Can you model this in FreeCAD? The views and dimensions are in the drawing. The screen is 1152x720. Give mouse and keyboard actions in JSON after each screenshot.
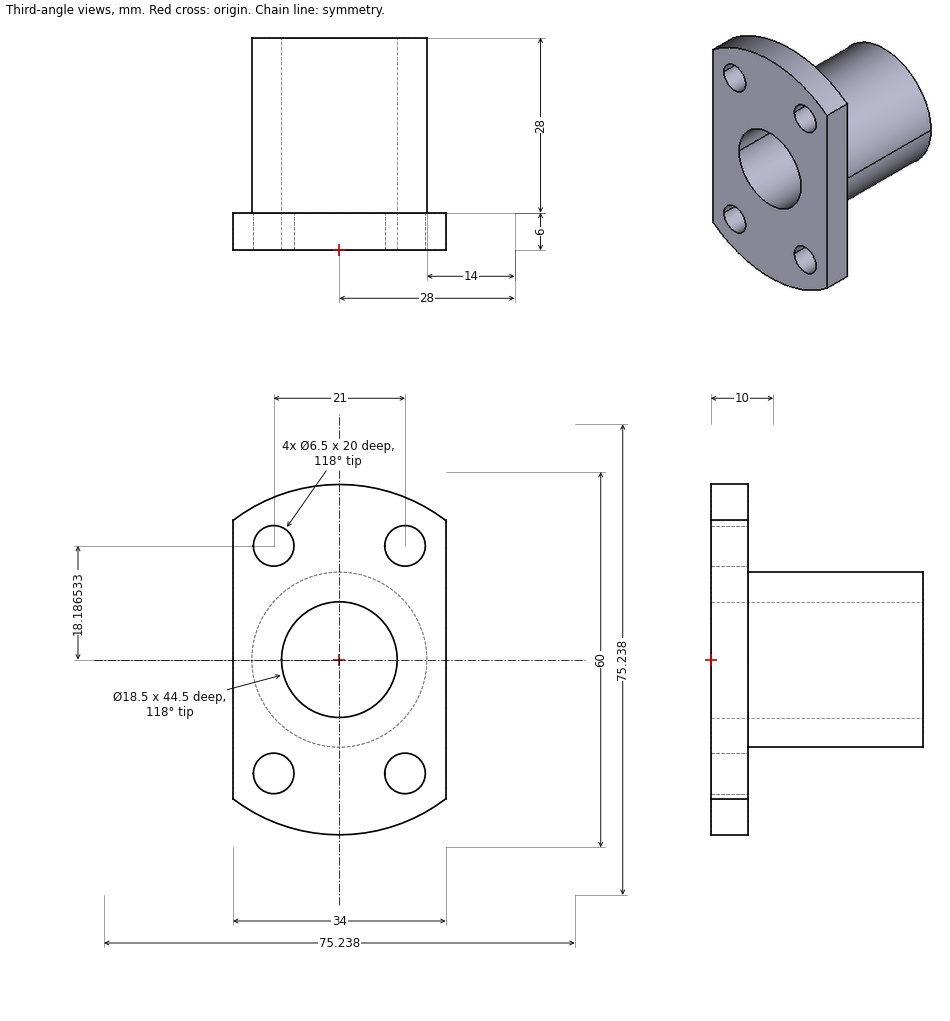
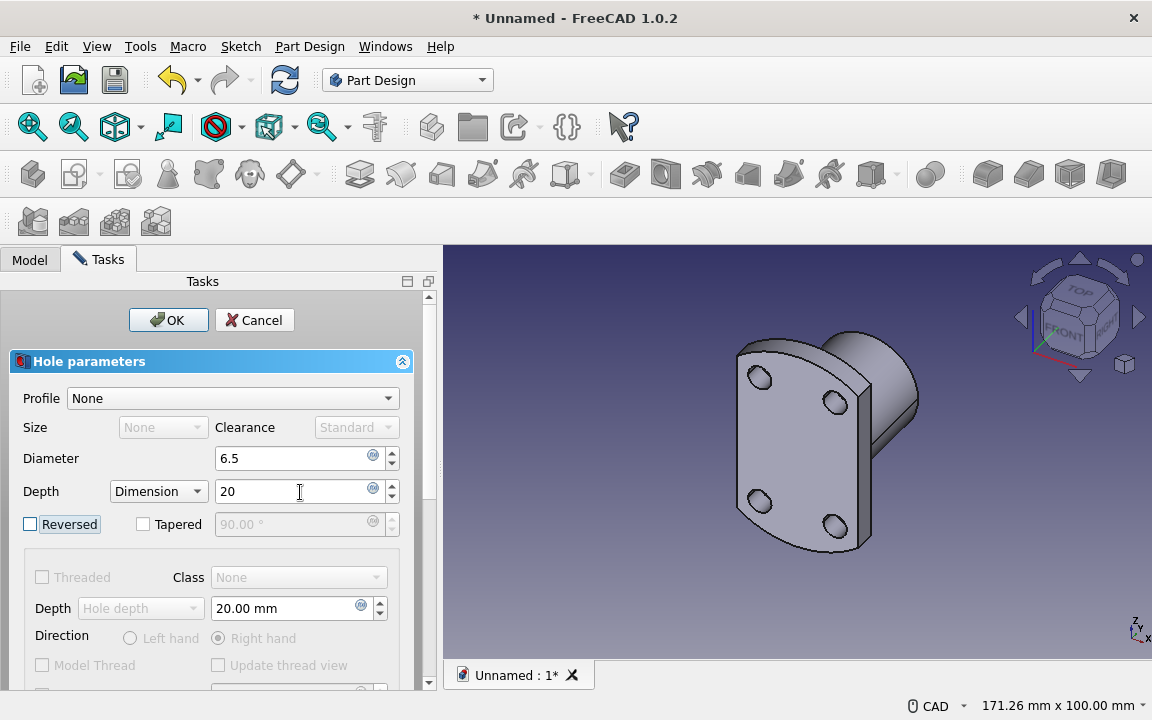
{"action": "left_click", "coordinate": [169, 320]}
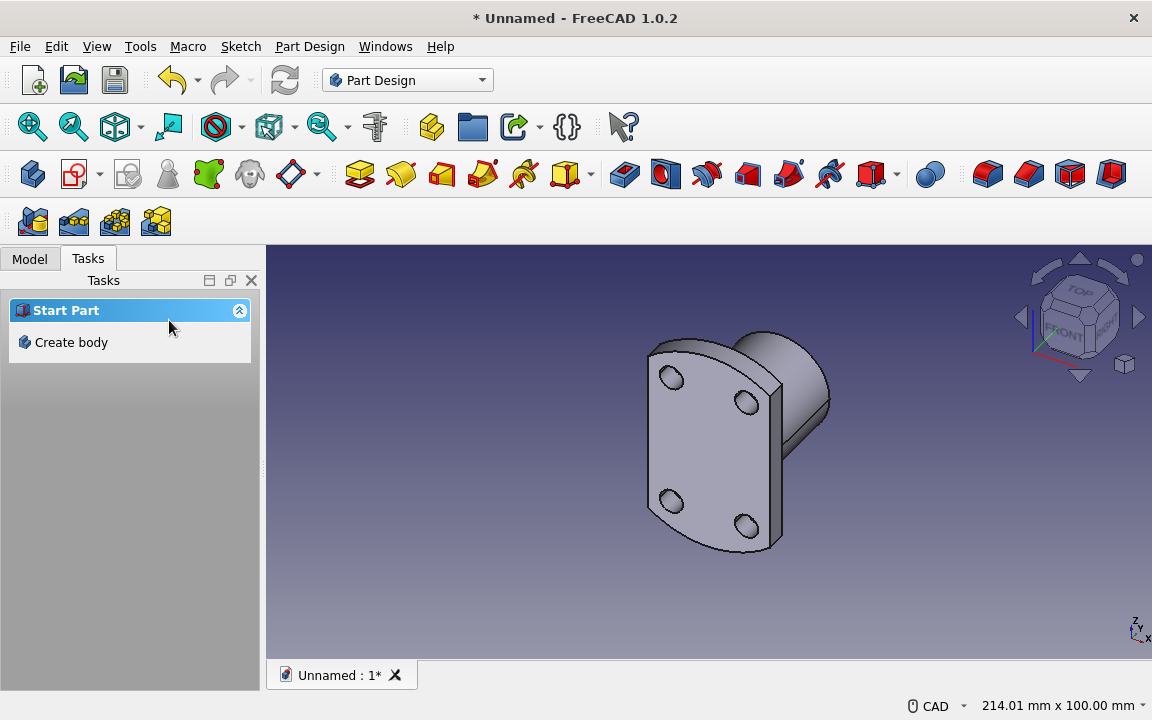
{"action": "left_click", "coordinate": [709, 451]}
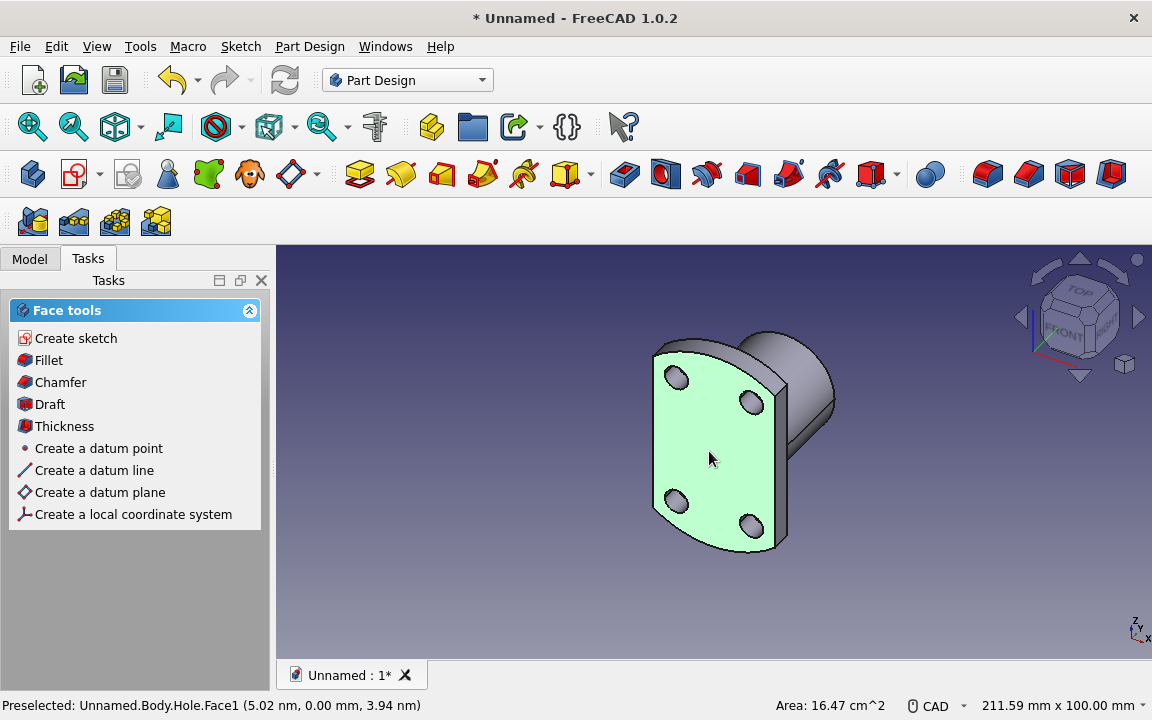
{"action": "left_click", "coordinate": [74, 174]}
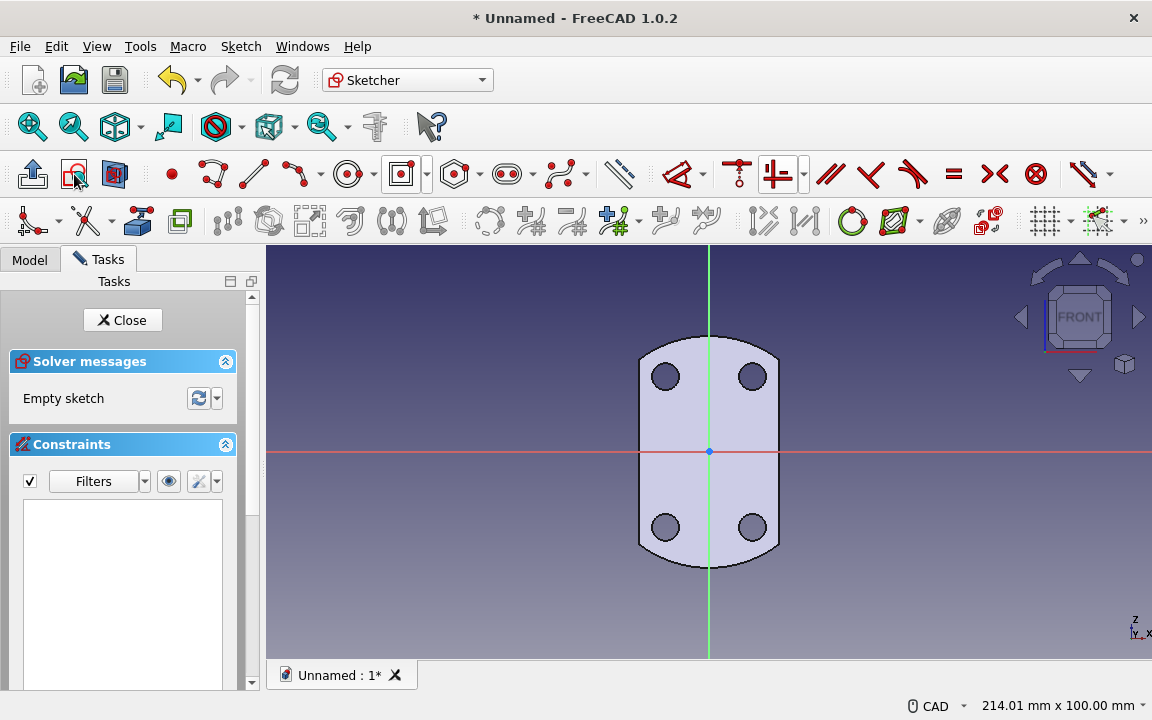
{"action": "scroll", "coordinate": [739, 452], "scroll_direction": "up", "scroll_amount": 6}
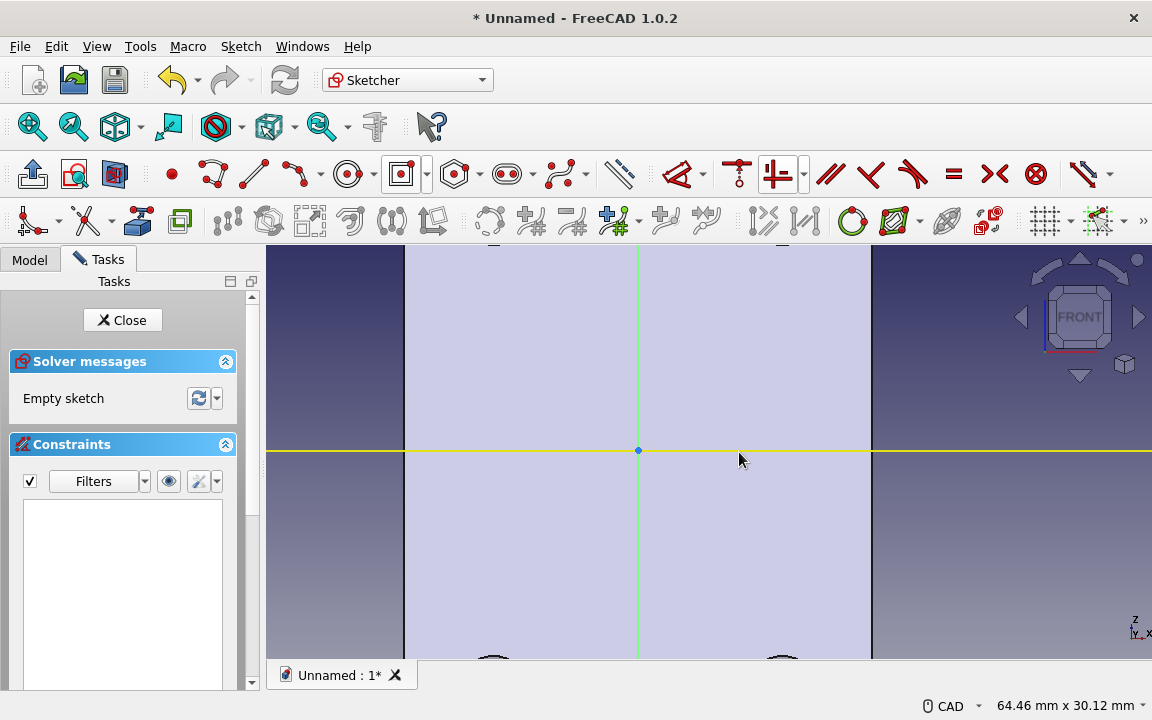
{"action": "left_click", "coordinate": [348, 174]}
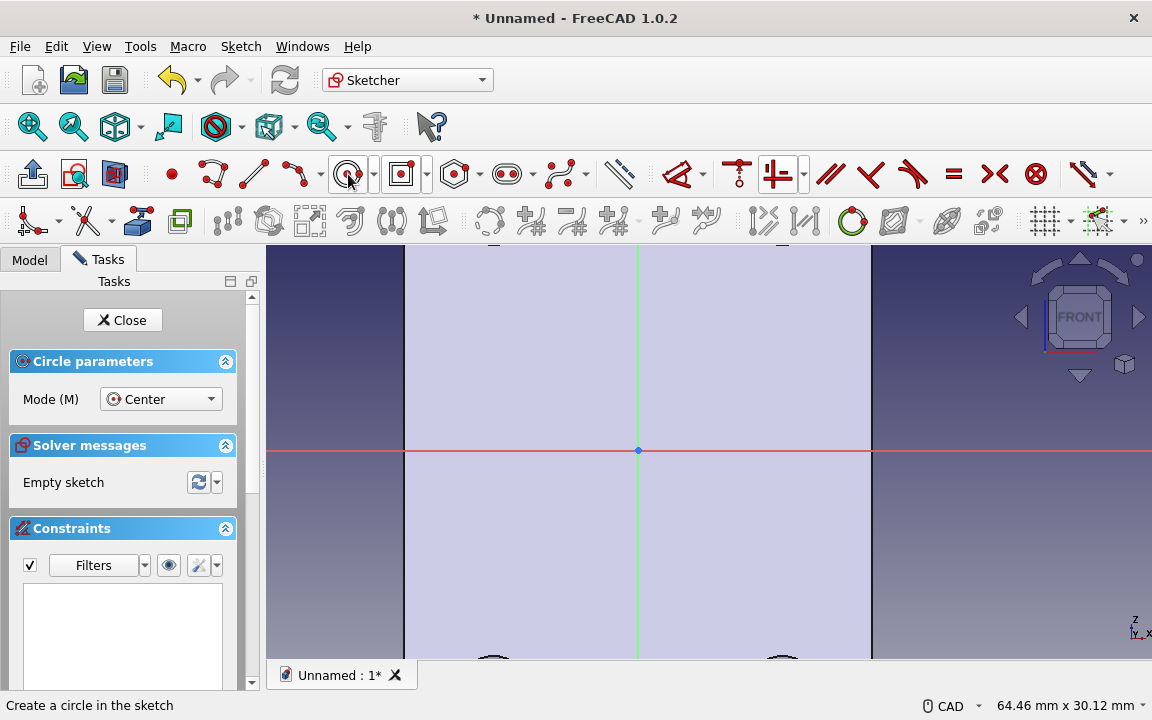
{"action": "left_click", "coordinate": [638, 451]}
{"action": "mouse_move", "coordinate": [728, 361]}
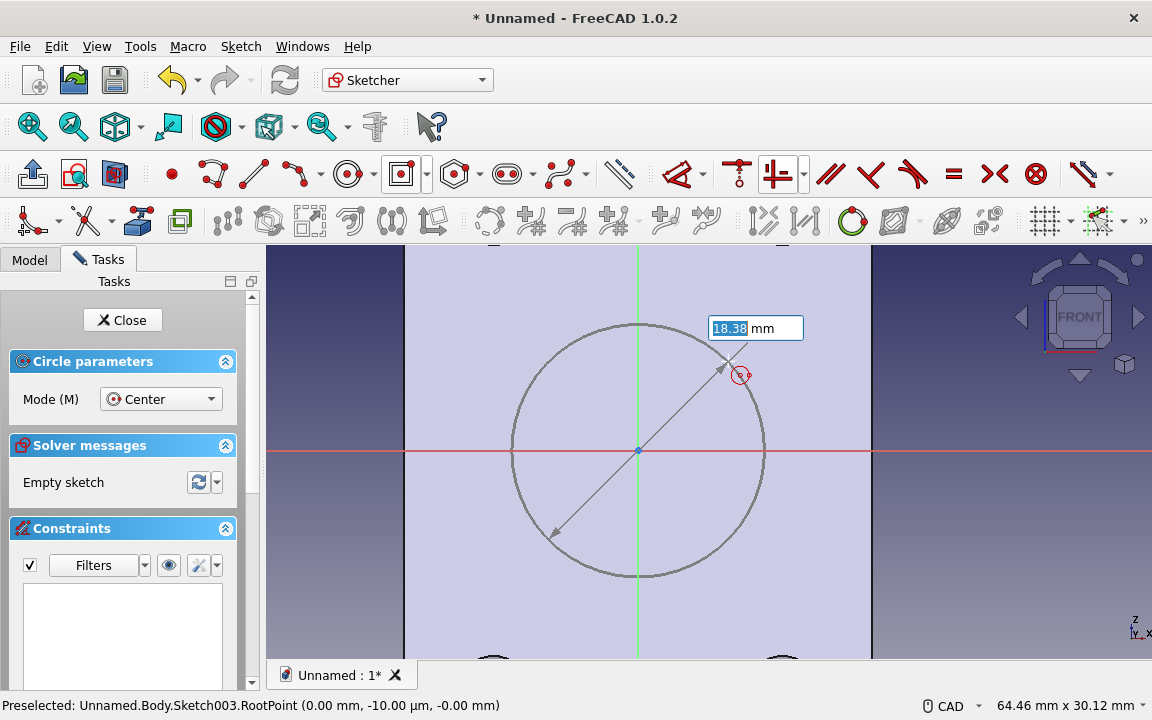
{"action": "type", "text": "18.5"}
{"action": "key", "text": "Return"}
{"action": "key", "text": "Escape"}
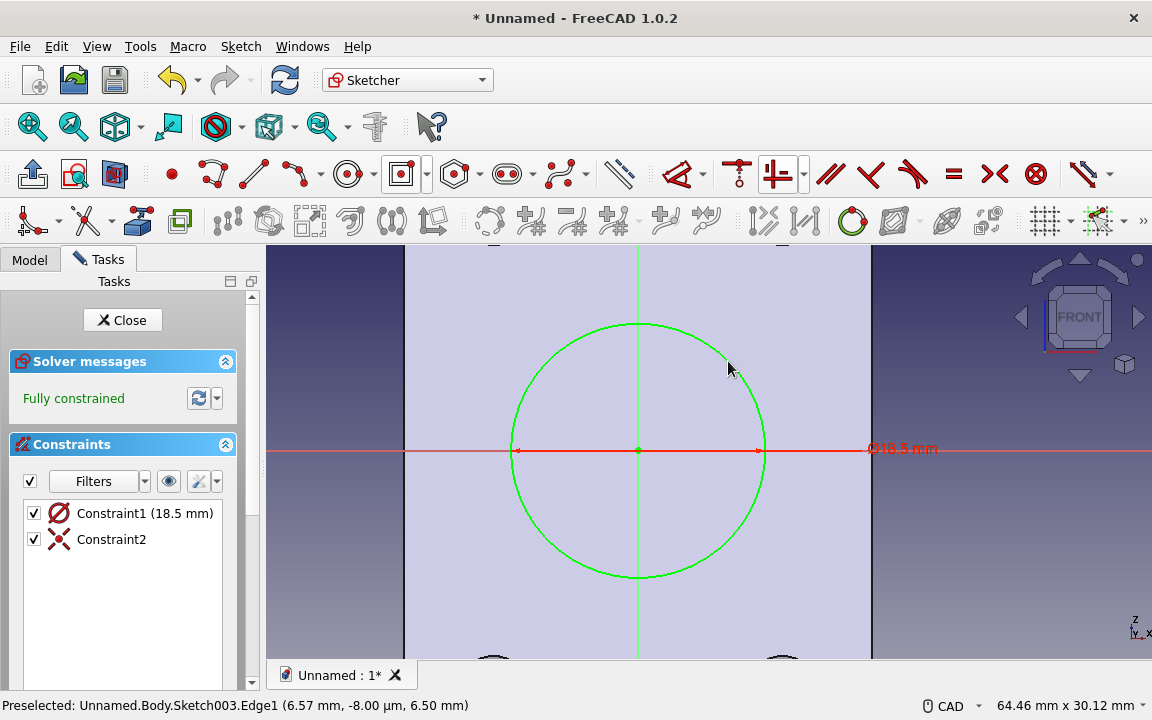
{"action": "left_click", "coordinate": [123, 320]}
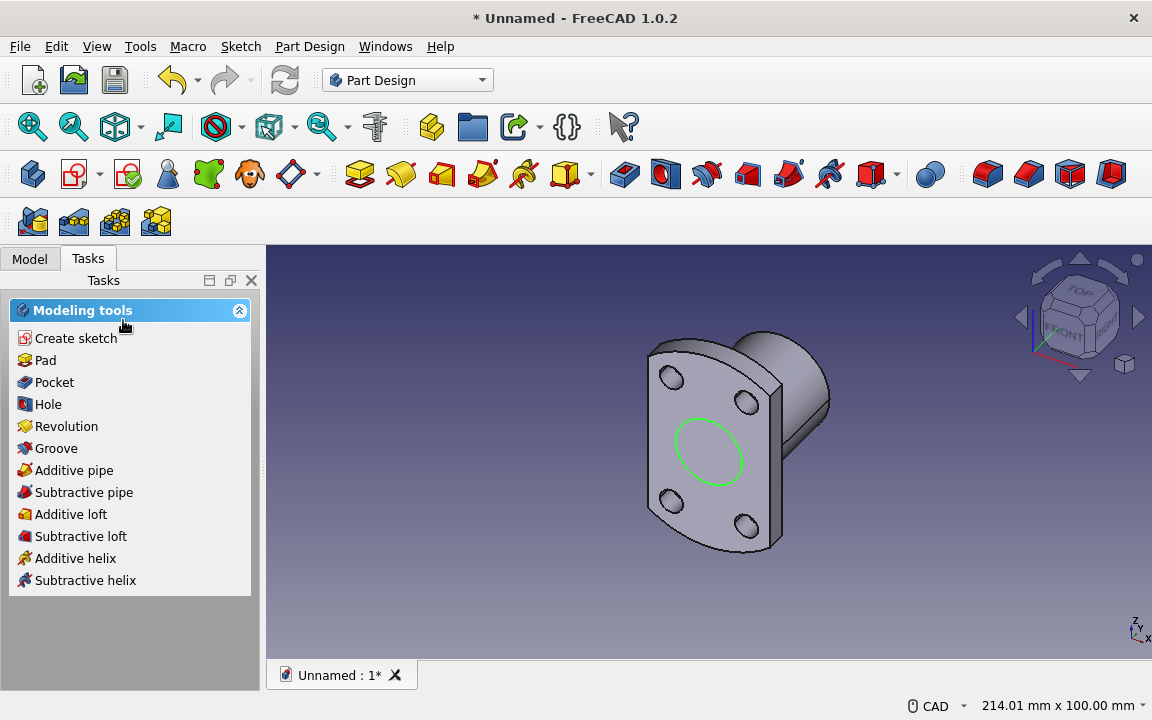
{"action": "left_click", "coordinate": [666, 174]}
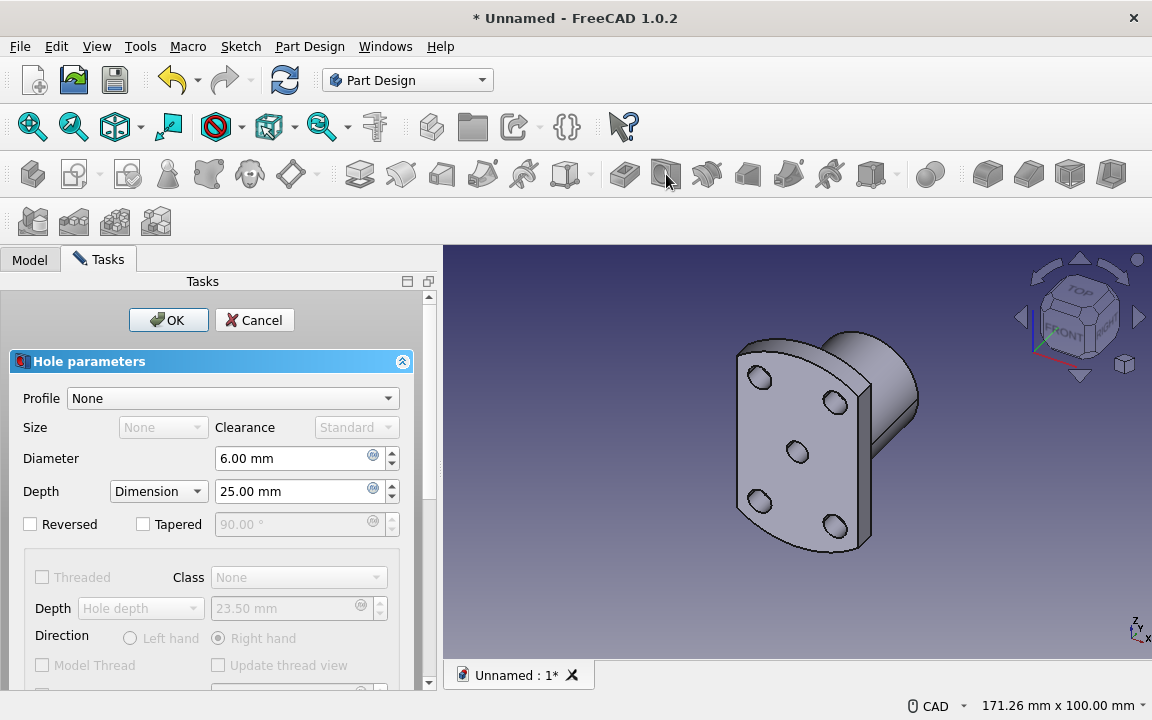
{"action": "triple_click", "coordinate": [300, 458]}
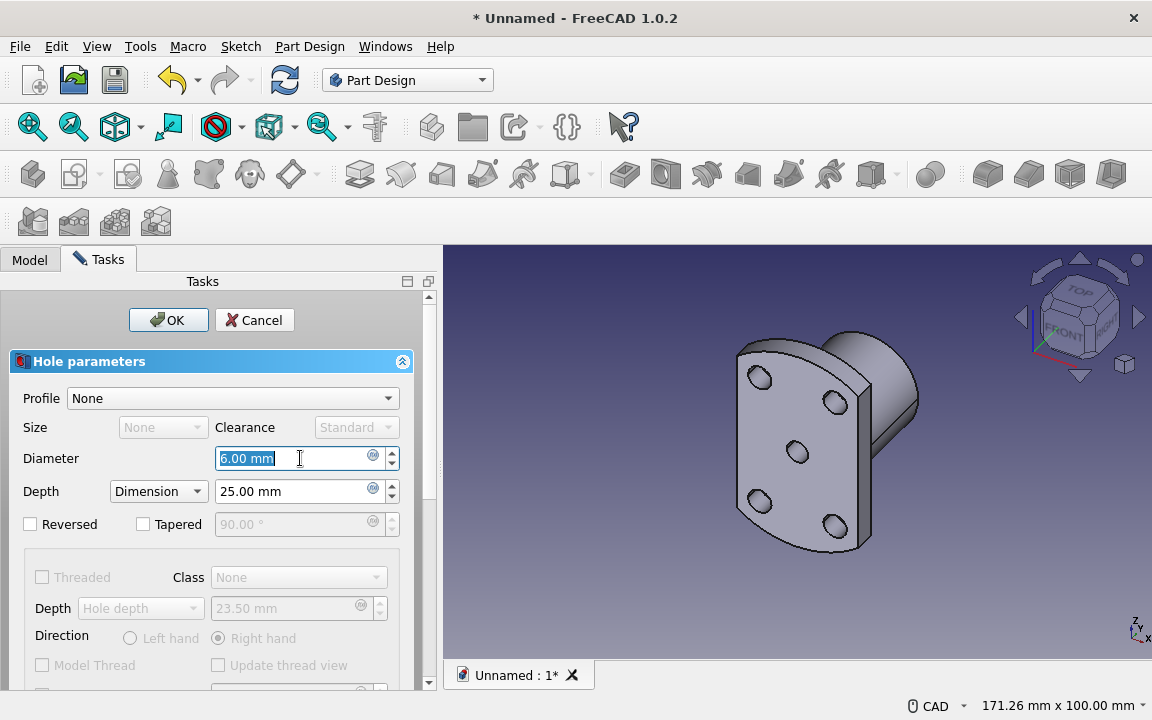
{"action": "type", "text": "18.5"}
{"action": "key", "text": "Tab"}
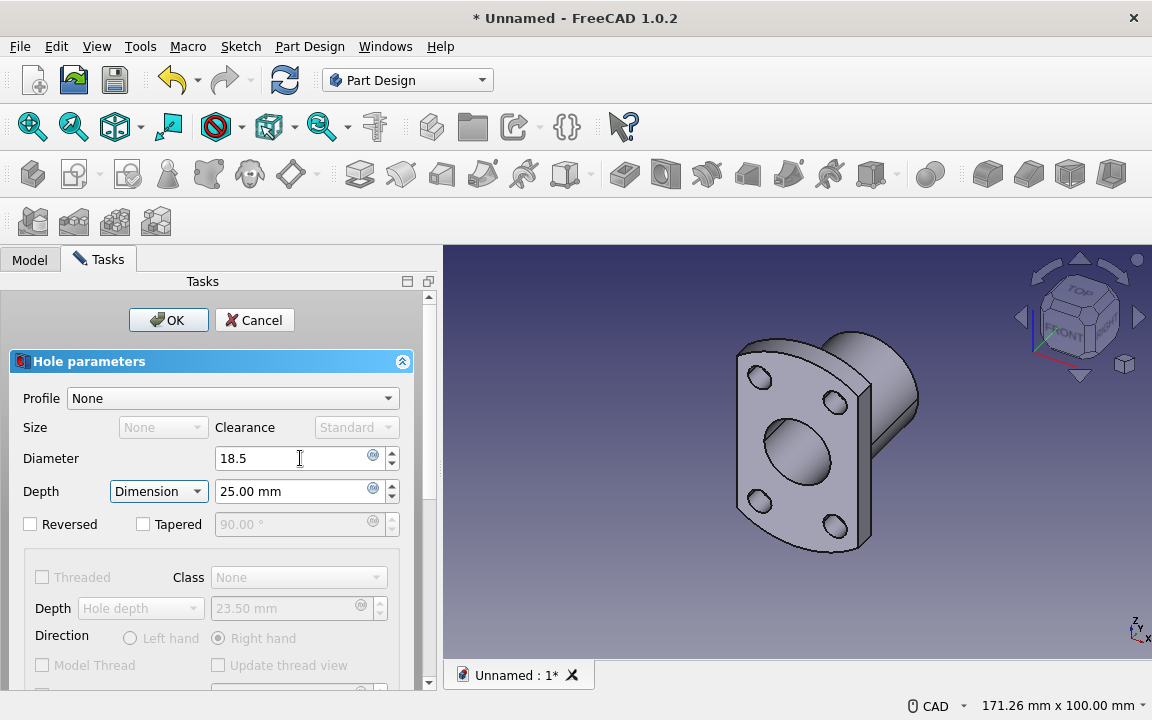
{"action": "triple_click", "coordinate": [300, 492]}